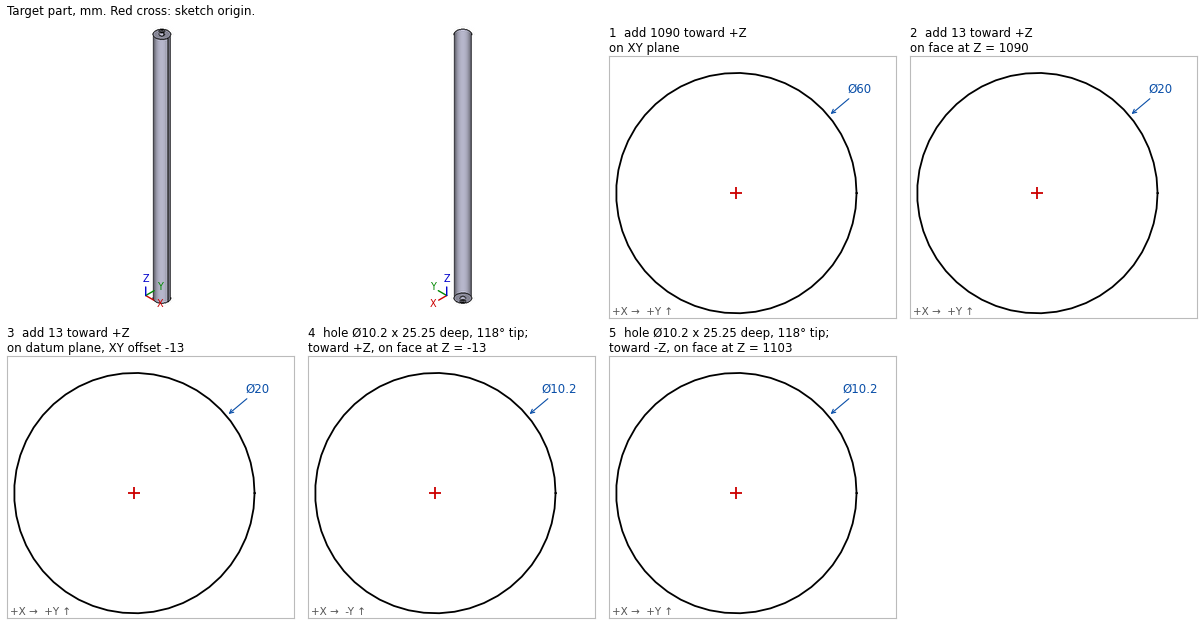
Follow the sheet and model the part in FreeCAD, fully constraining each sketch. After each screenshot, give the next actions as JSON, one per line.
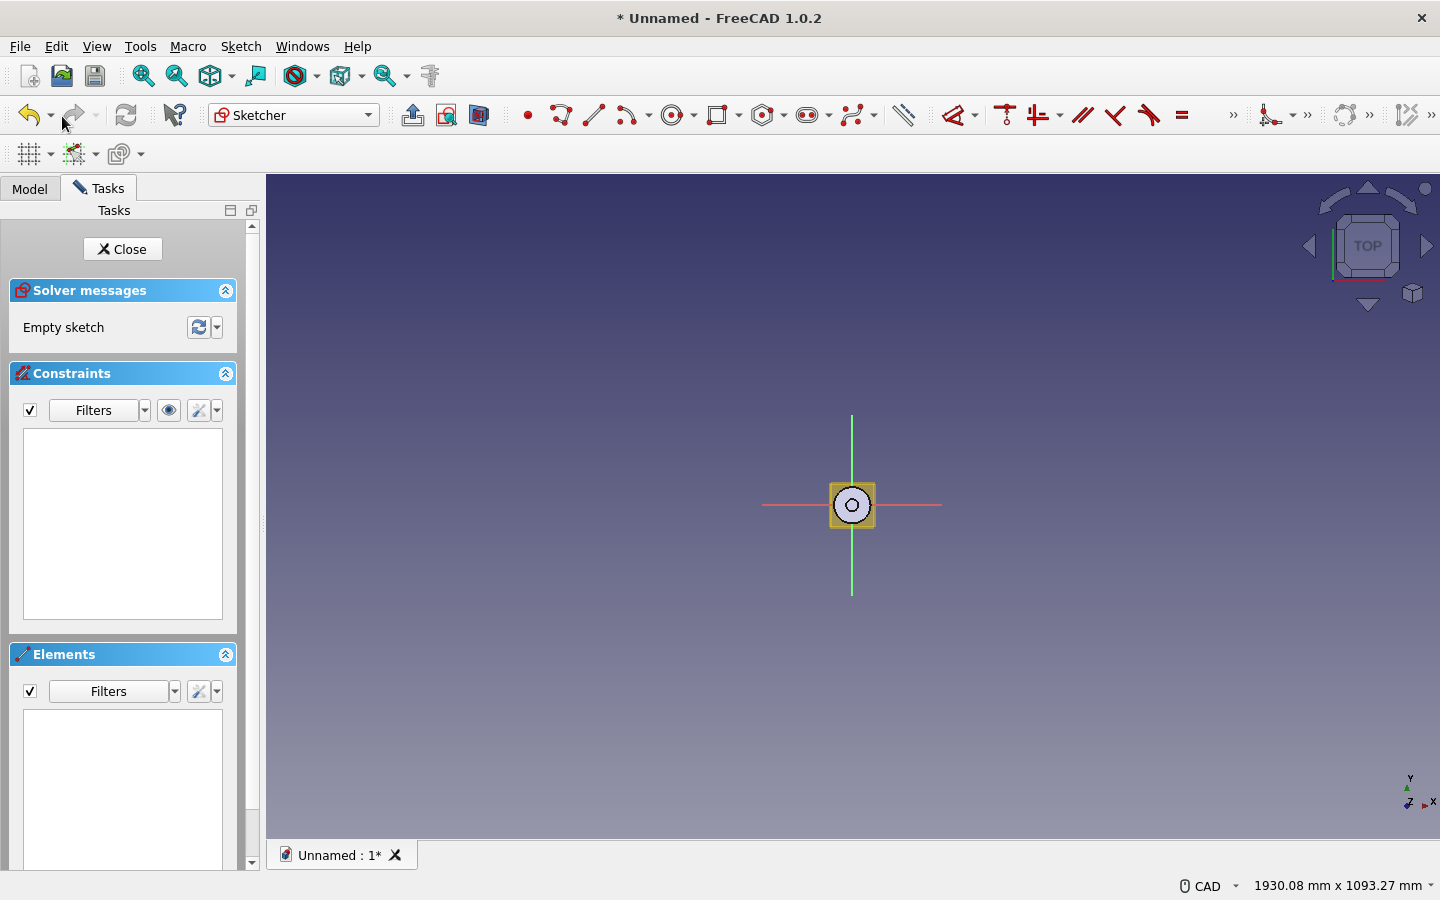
{"action": "key", "text": "q s"}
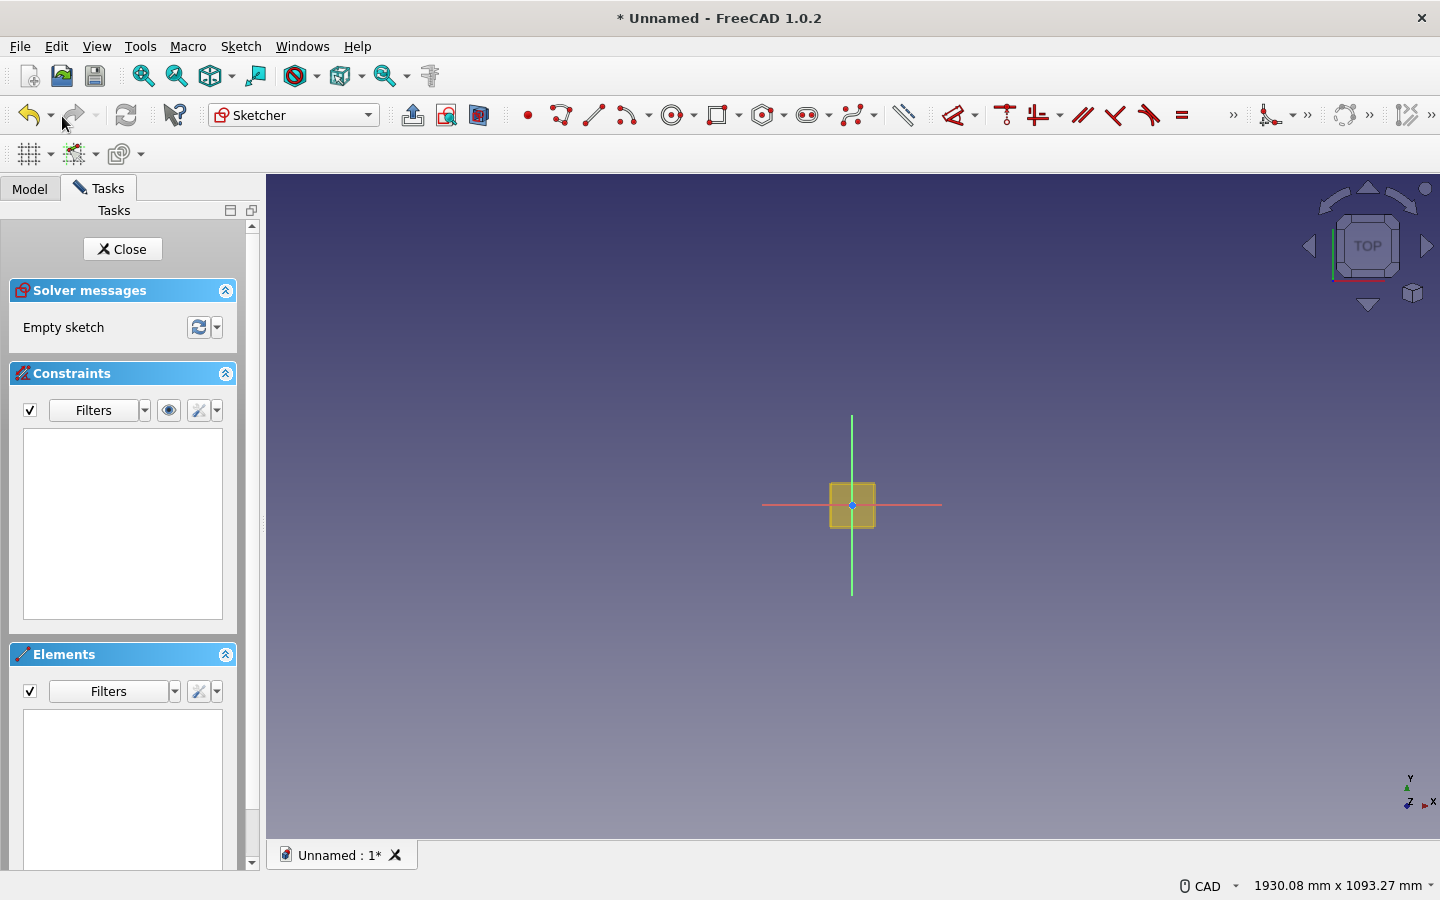
{"action": "scroll", "coordinate": [856, 505], "scroll_direction": "up", "scroll_amount": 15}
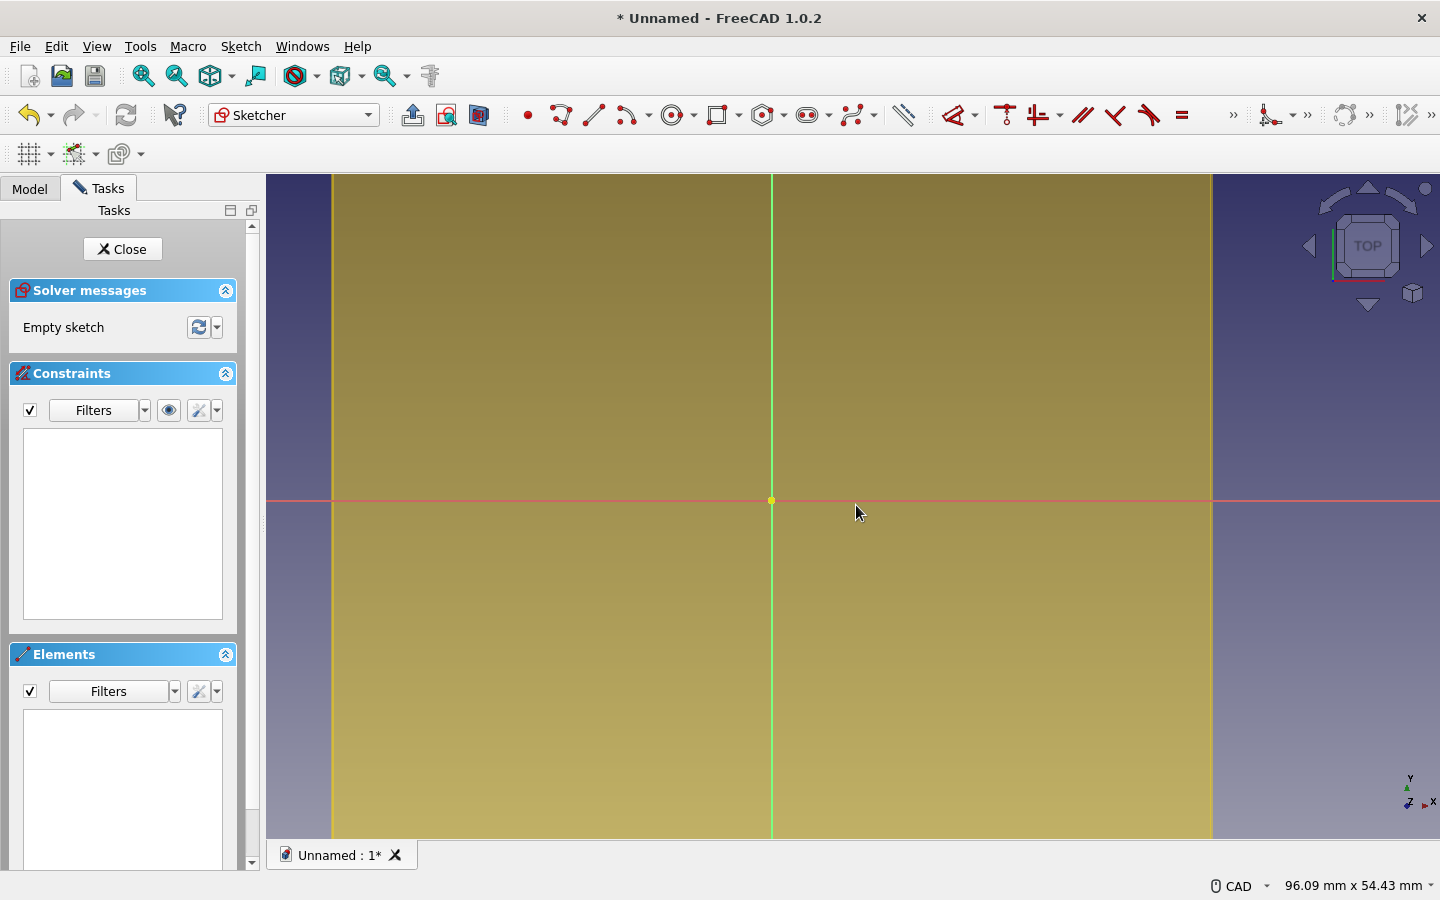
{"action": "scroll", "coordinate": [756, 493], "scroll_direction": "up", "scroll_amount": 3}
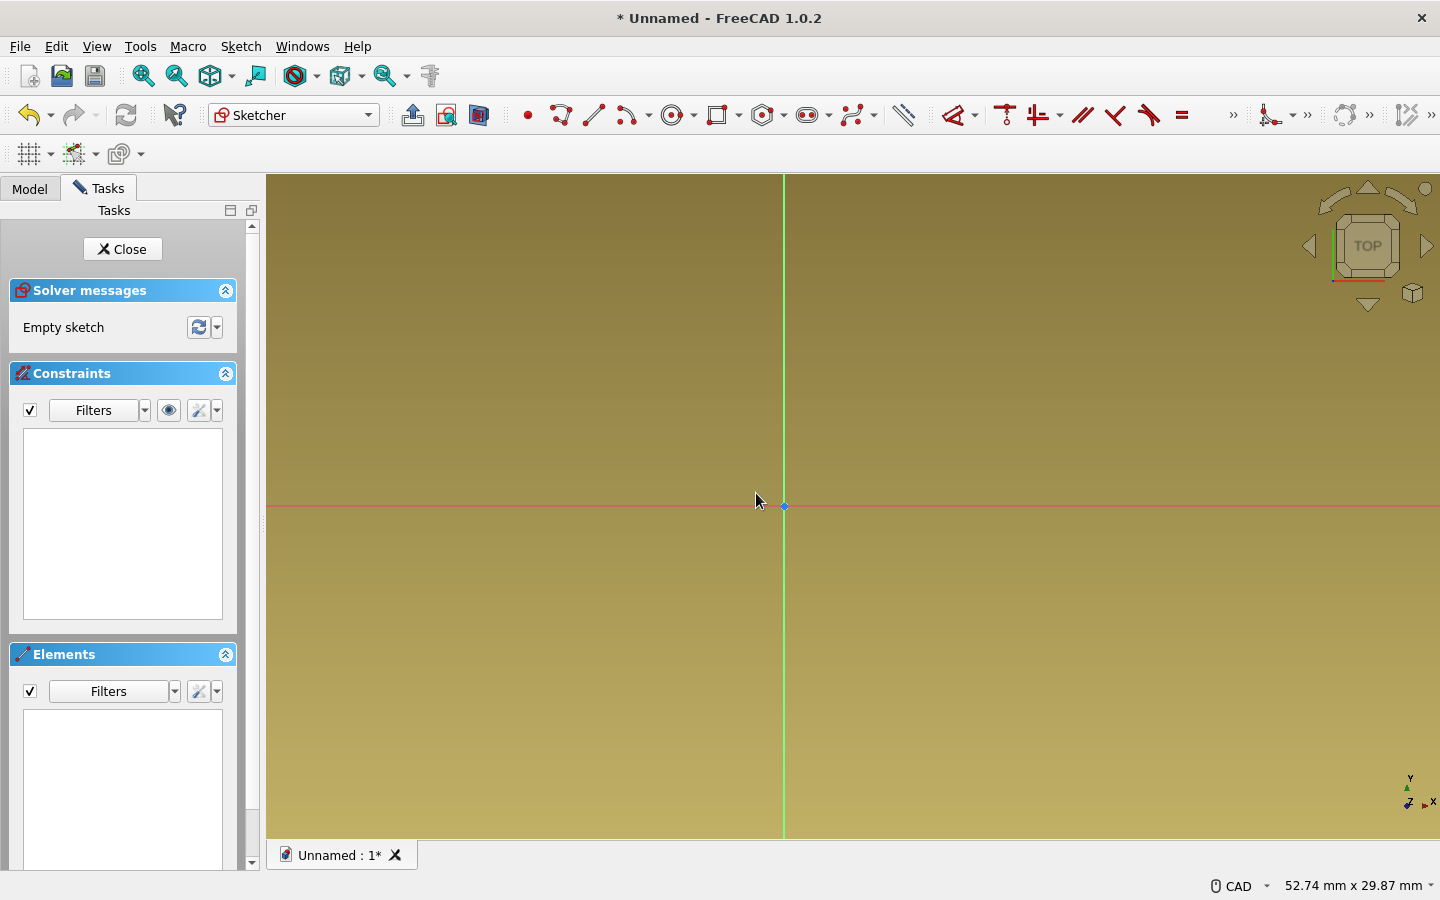
{"action": "left_click", "coordinate": [672, 116]}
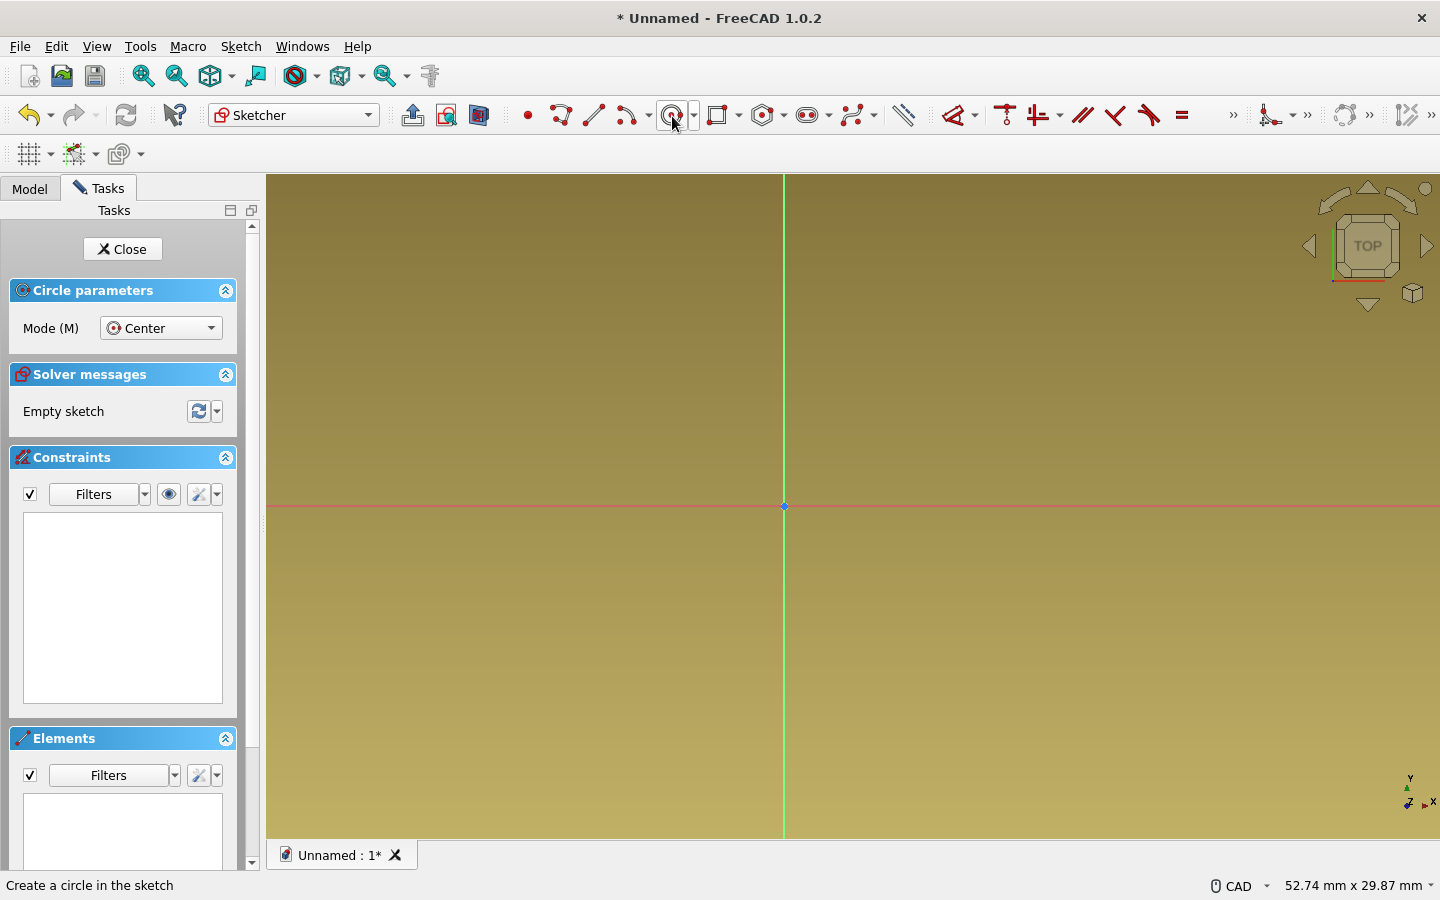
{"action": "left_click", "coordinate": [784, 506]}
{"action": "mouse_move", "coordinate": [942, 349]}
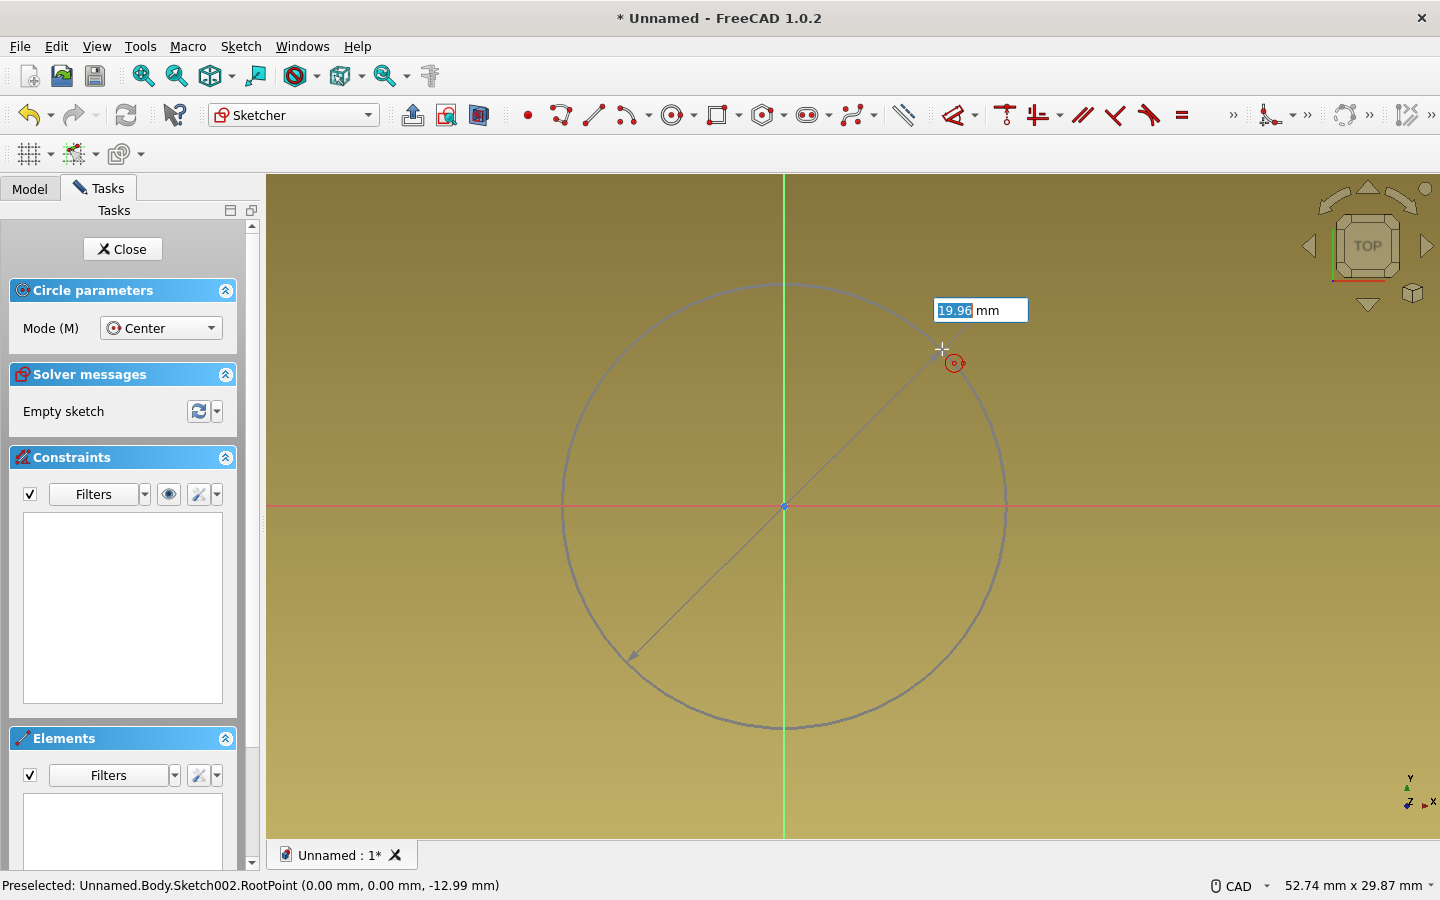
{"action": "type", "text": "20"}
{"action": "key", "text": "Return"}
{"action": "key", "text": "Escape"}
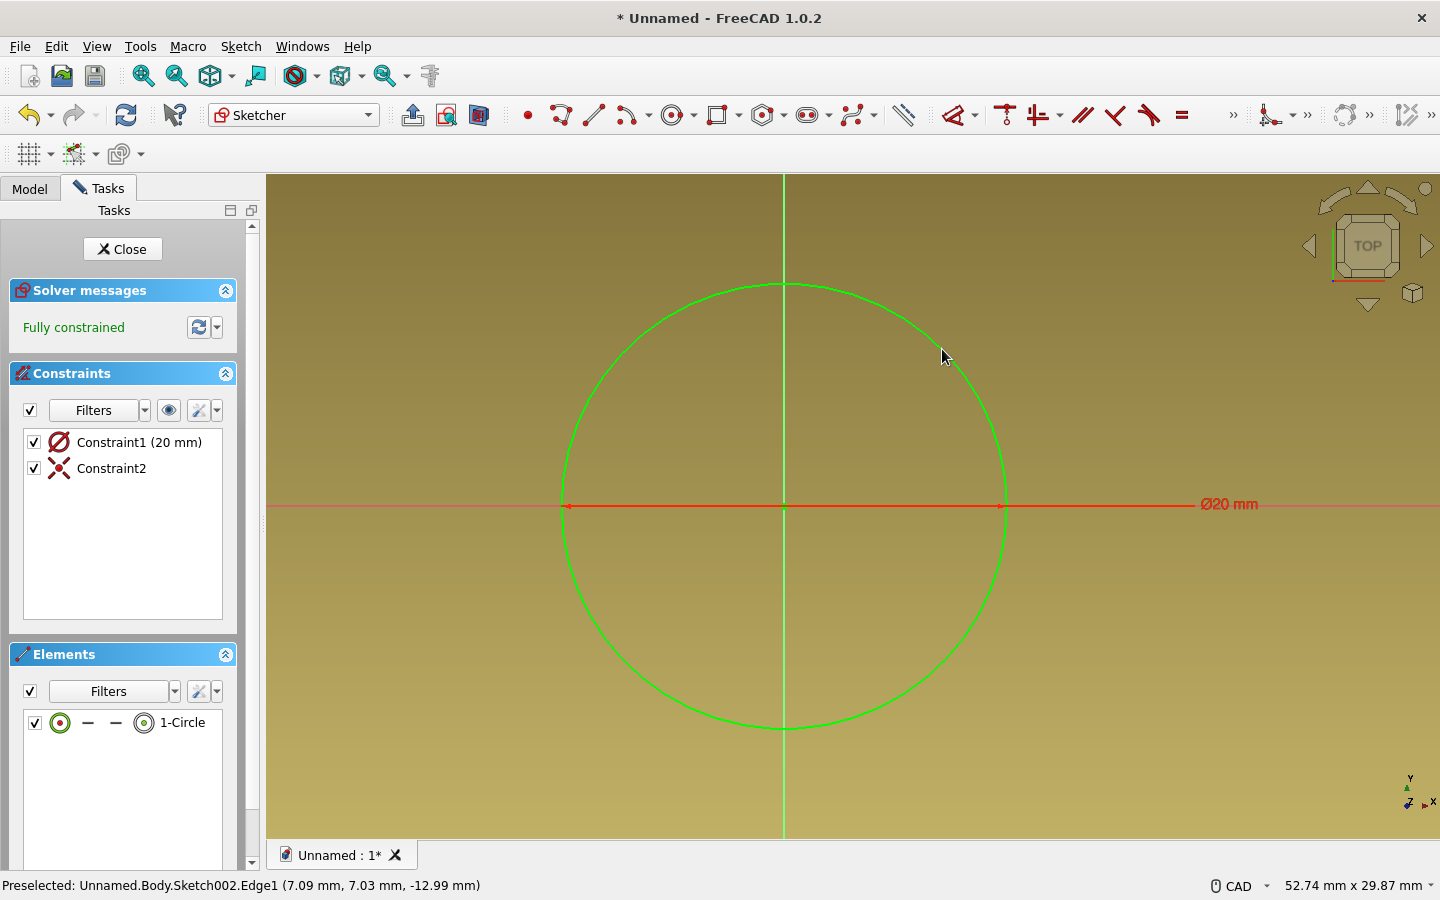
{"action": "left_click", "coordinate": [123, 249]}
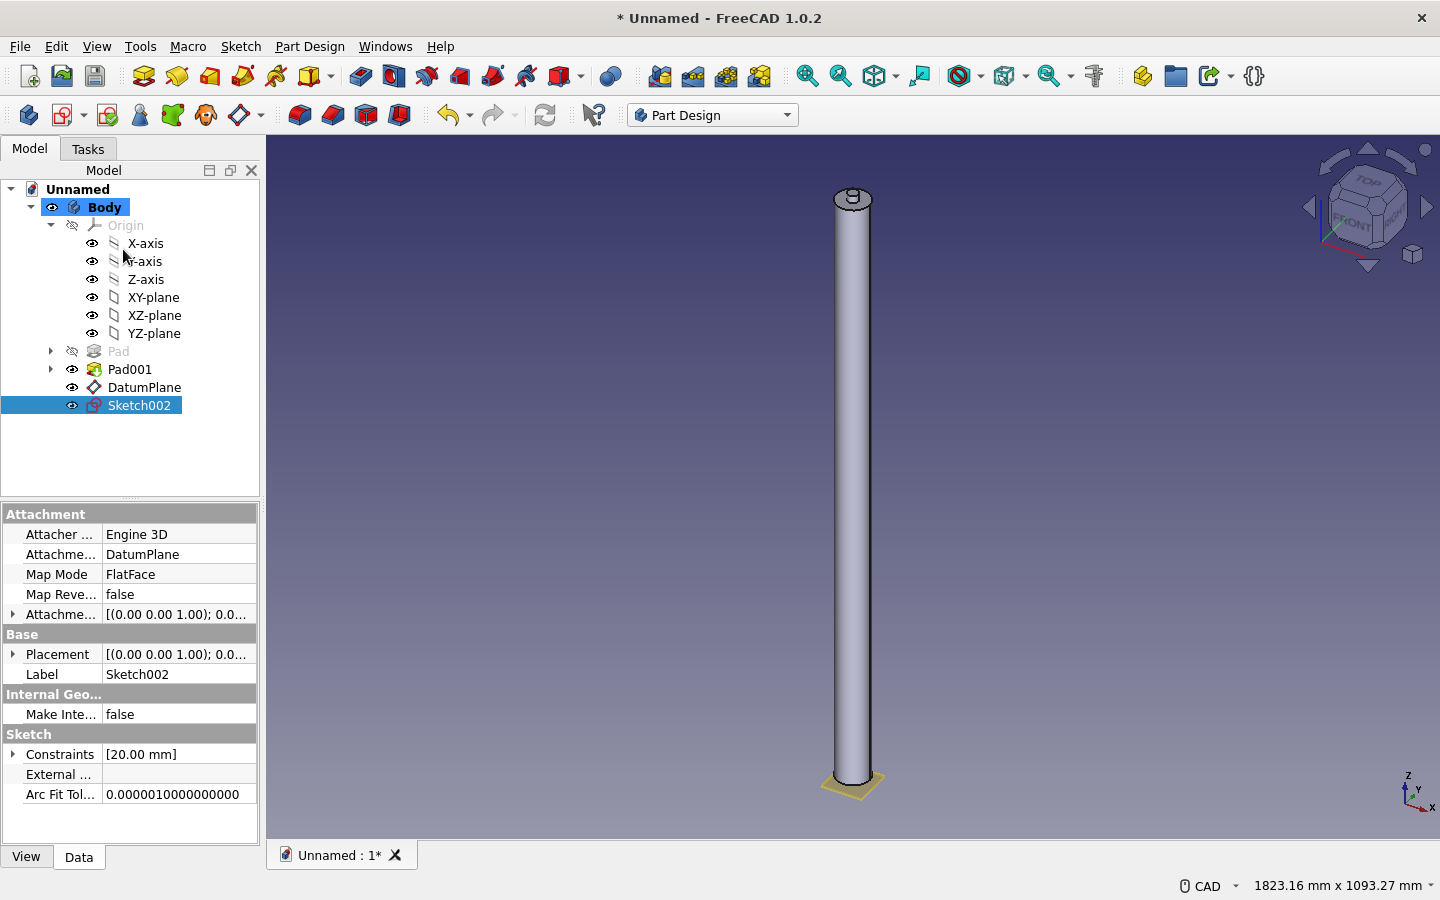
{"action": "left_click", "coordinate": [144, 76]}